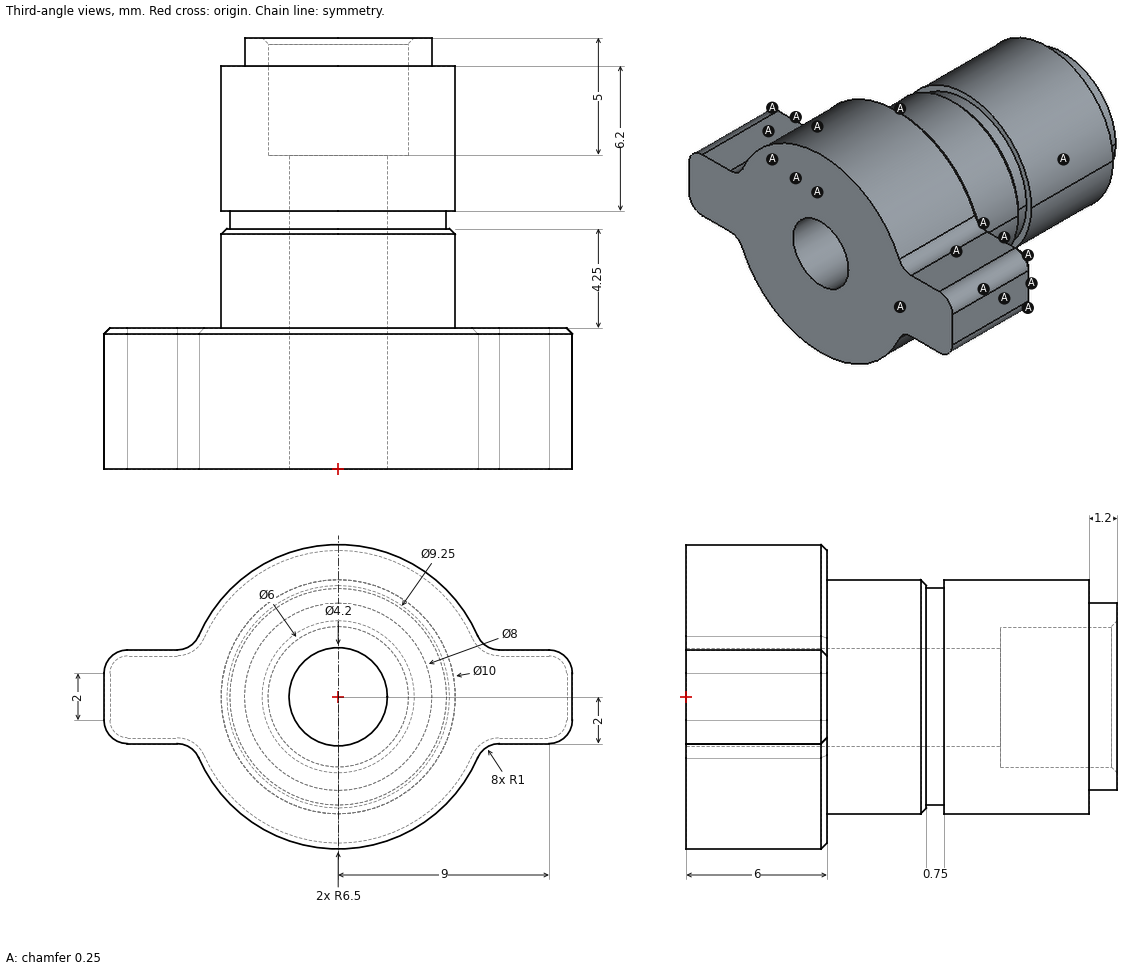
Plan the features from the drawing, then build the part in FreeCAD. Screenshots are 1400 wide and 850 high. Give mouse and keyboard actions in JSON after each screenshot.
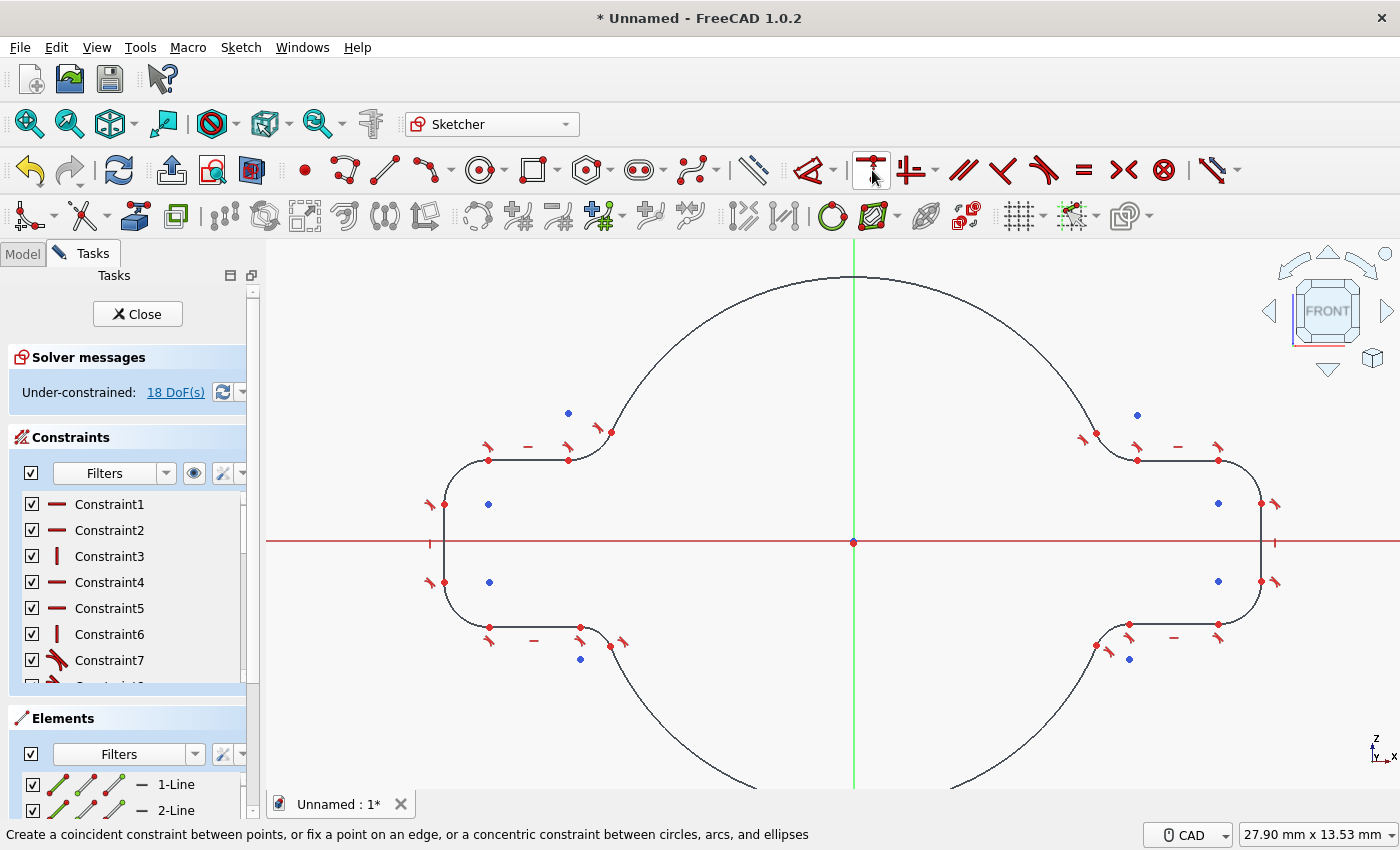
{"action": "scroll", "coordinate": [854, 542], "scroll_direction": "up", "scroll_amount": 2}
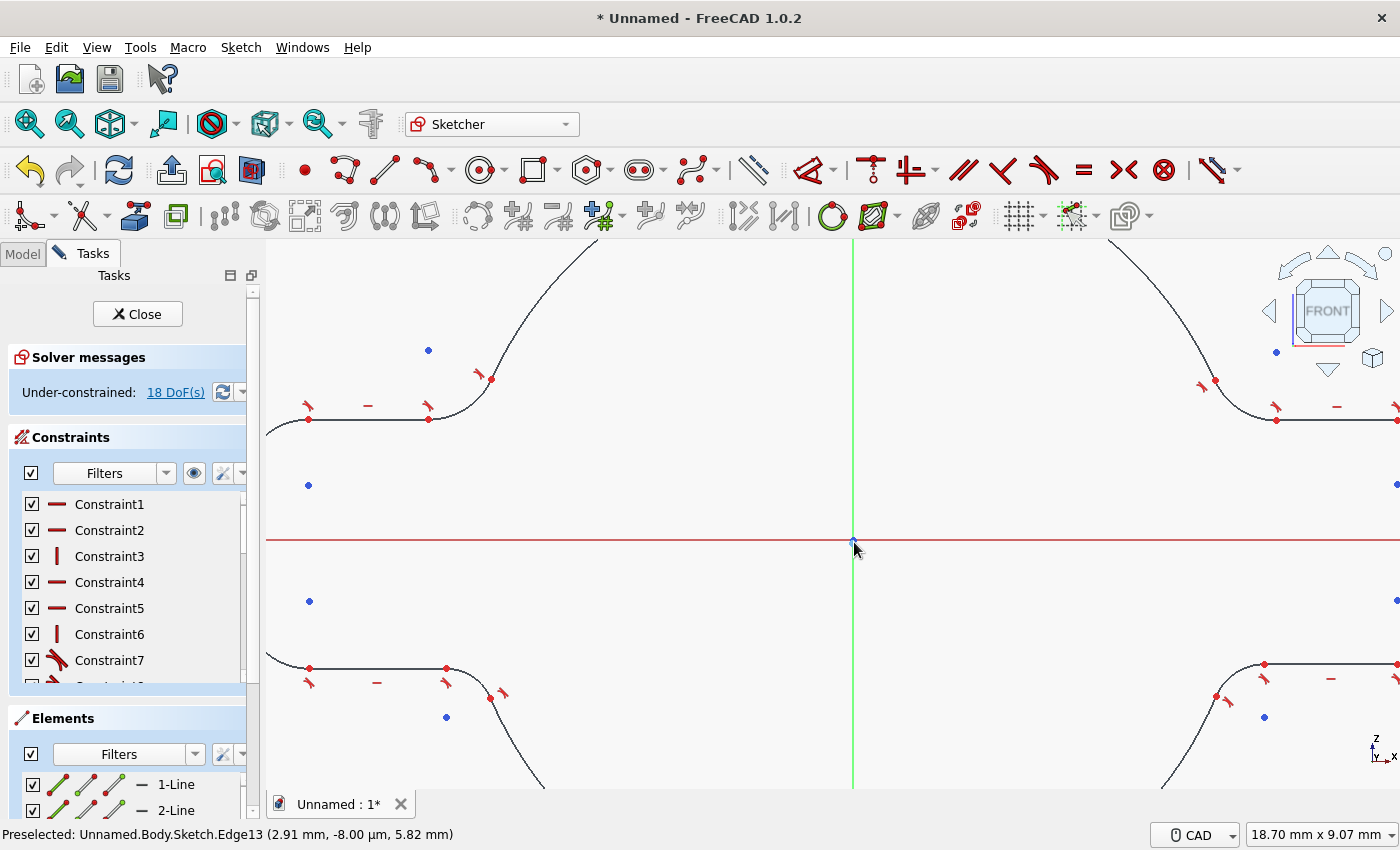
{"action": "left_click_drag", "start_coordinate": [843, 530], "coordinate": [863, 554]}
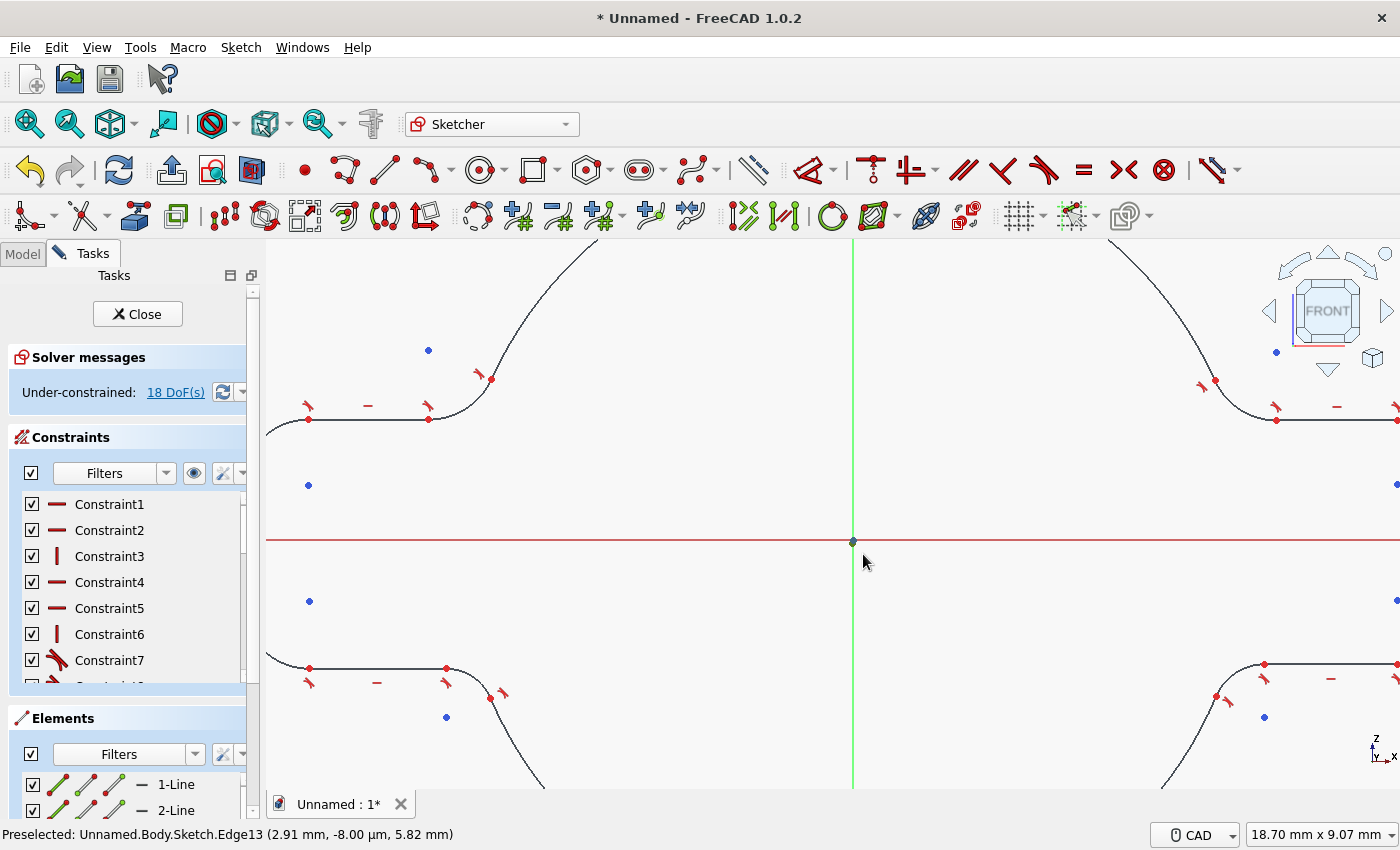
{"action": "left_click", "coordinate": [872, 170]}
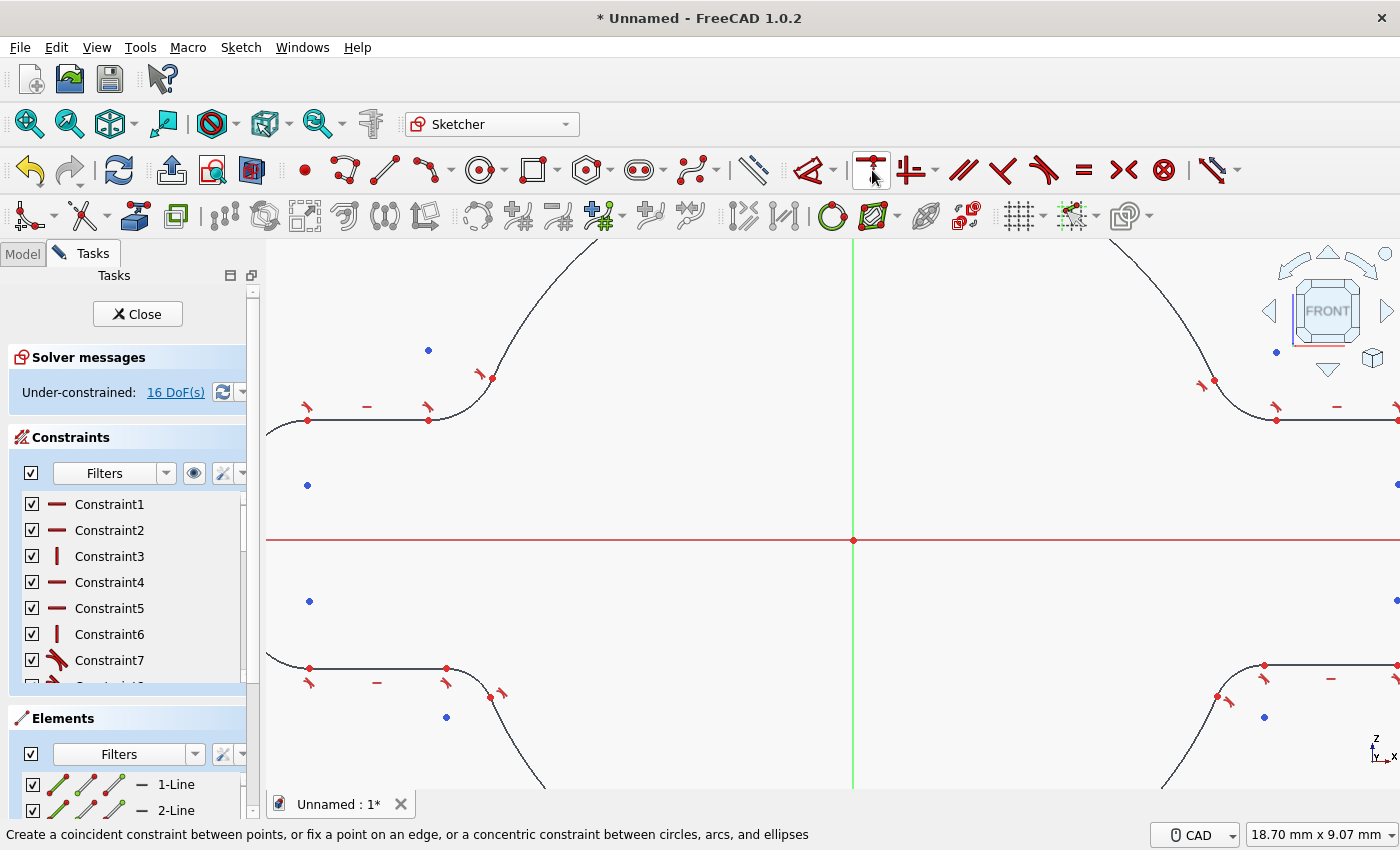
{"action": "left_click", "coordinate": [1227, 681]}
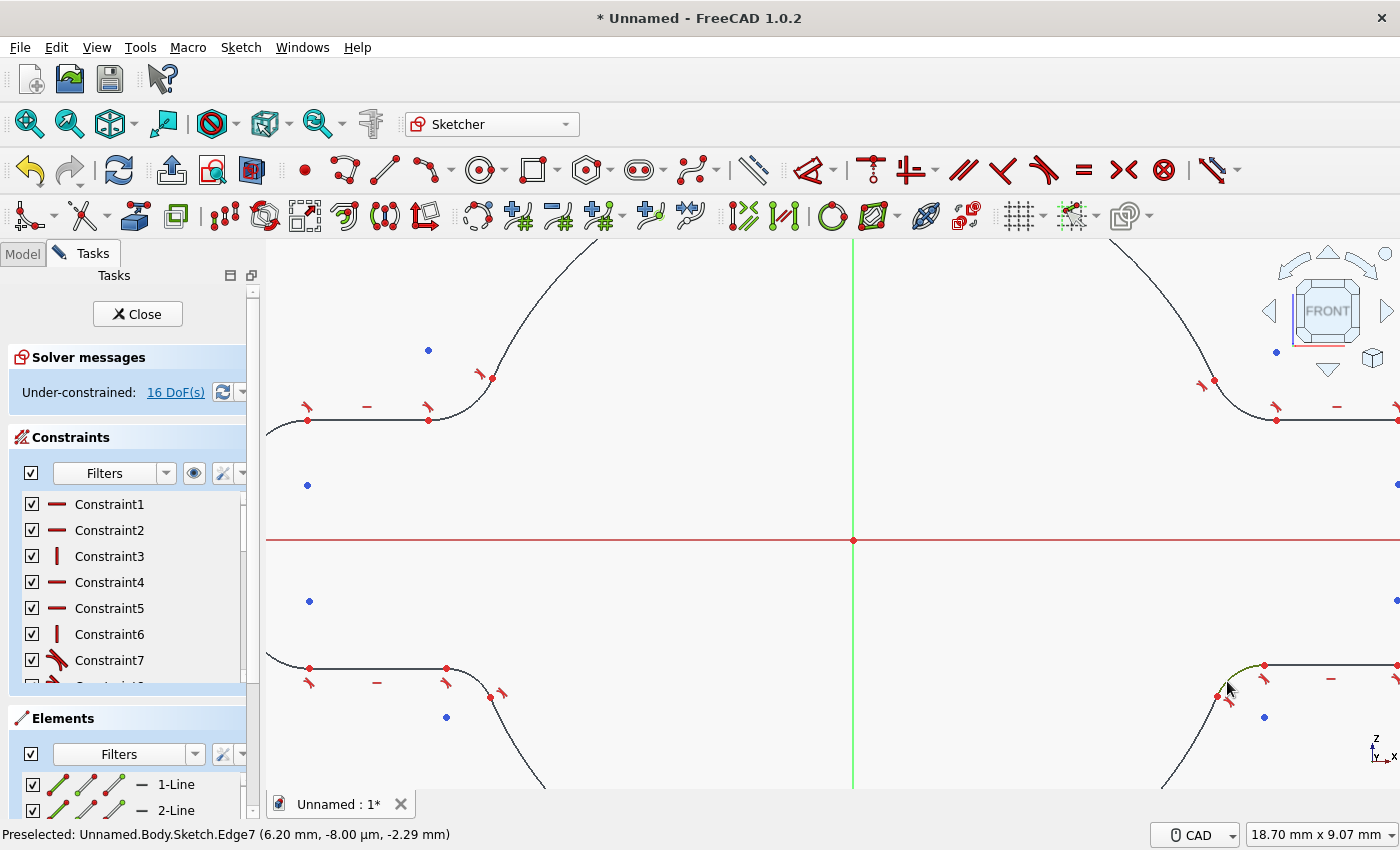
{"action": "left_click", "coordinate": [481, 684]}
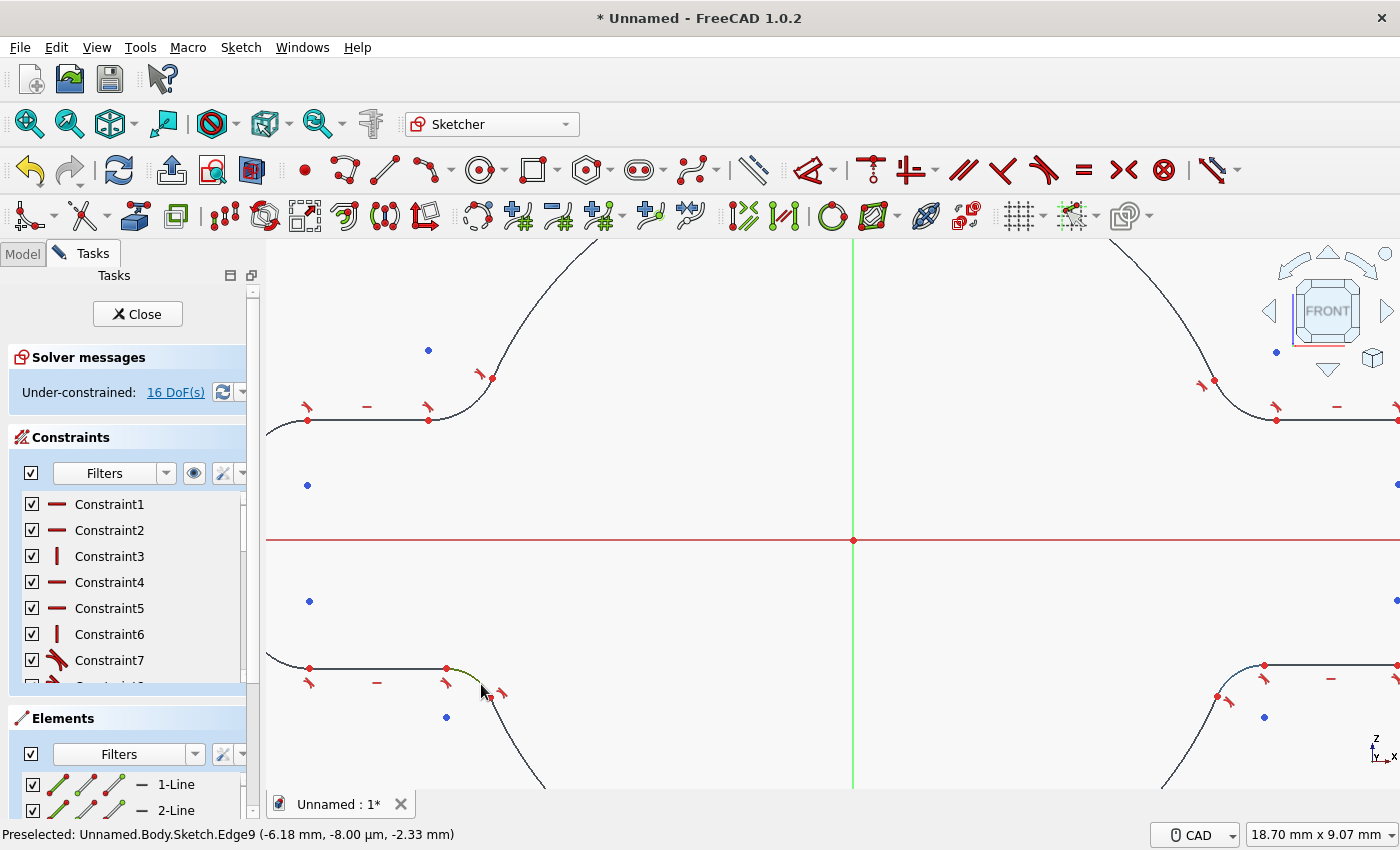
{"action": "scroll", "coordinate": [692, 493], "scroll_direction": "down", "scroll_amount": 4}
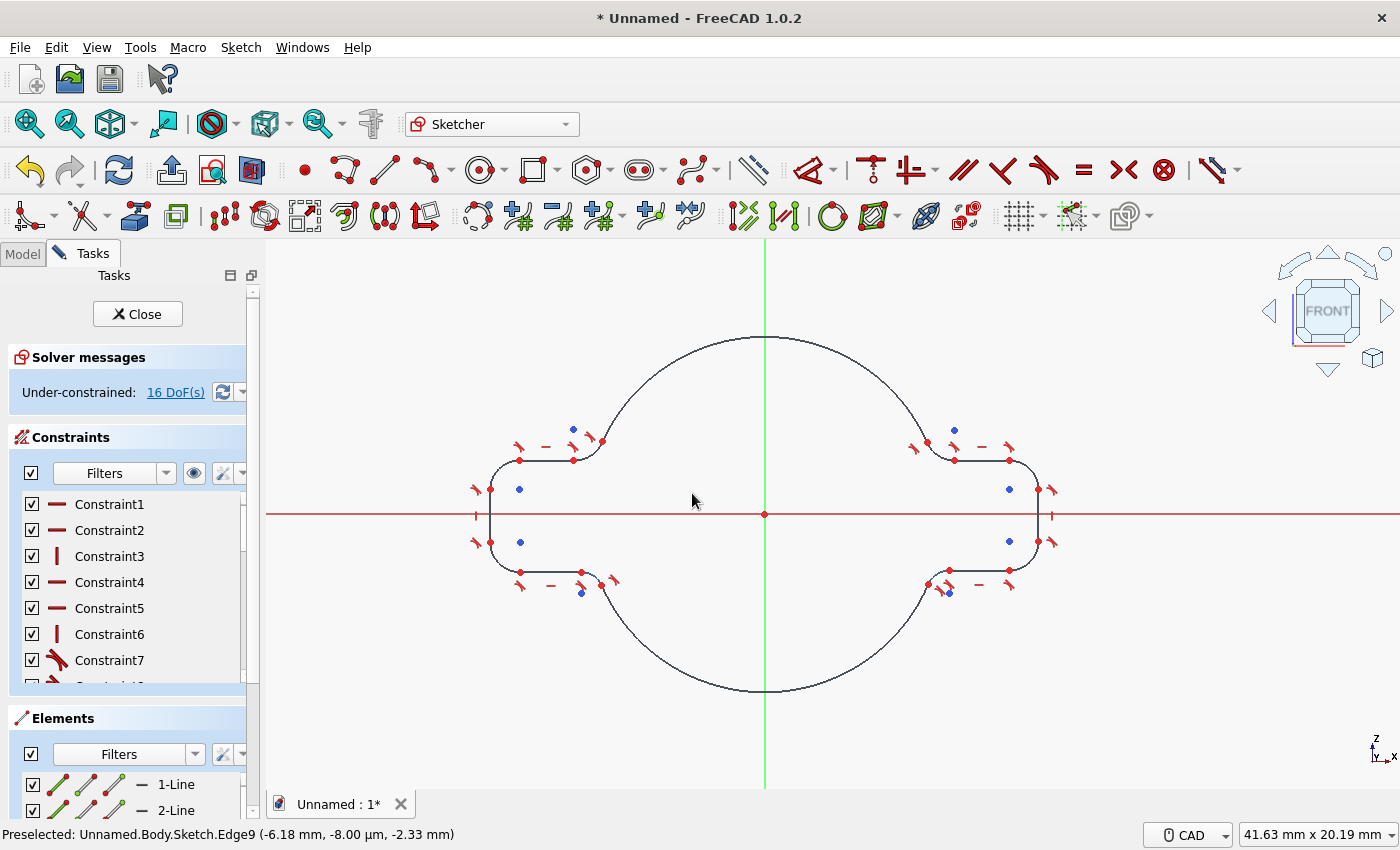
{"action": "left_click", "coordinate": [494, 556]}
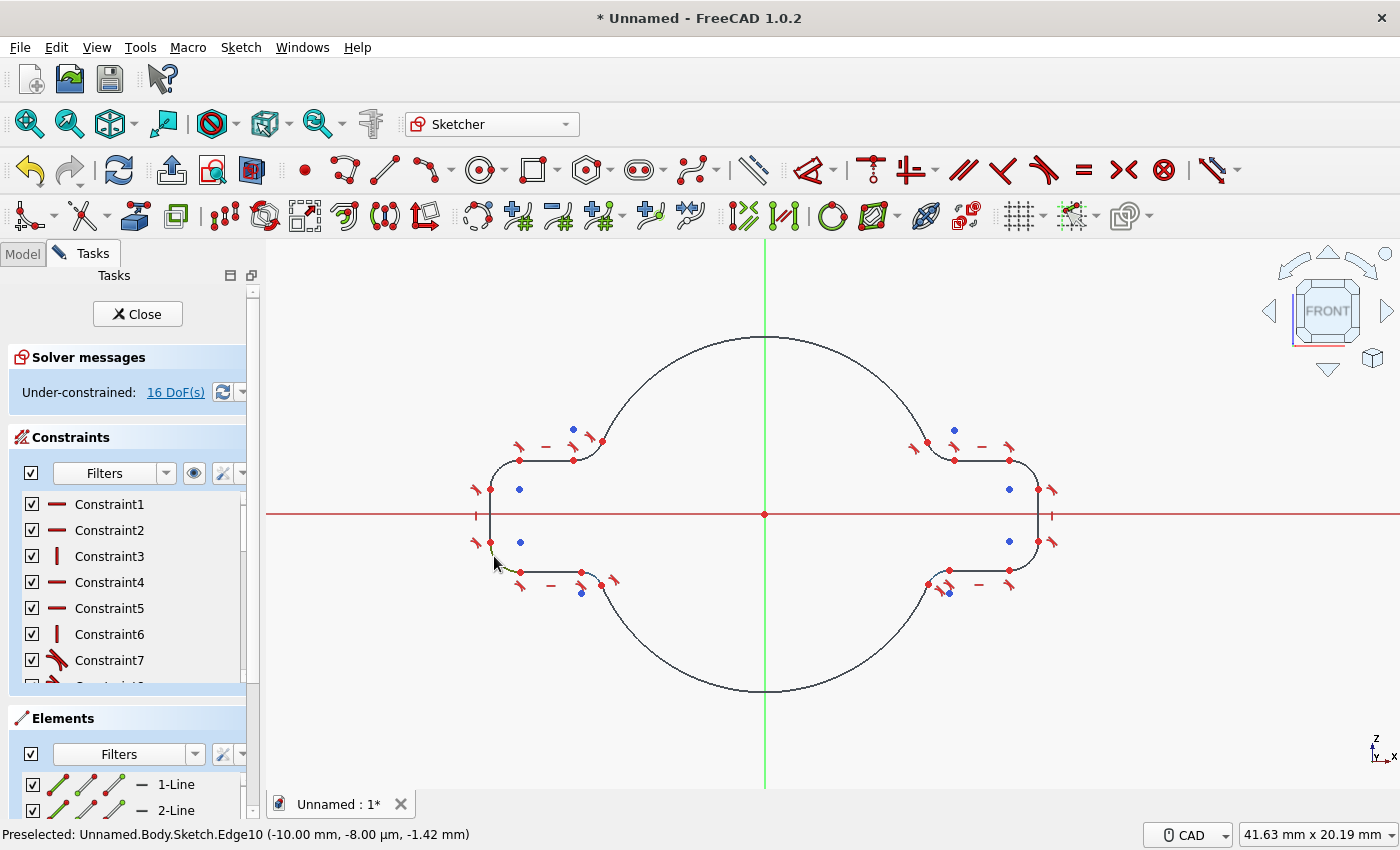
{"action": "left_click", "coordinate": [506, 464]}